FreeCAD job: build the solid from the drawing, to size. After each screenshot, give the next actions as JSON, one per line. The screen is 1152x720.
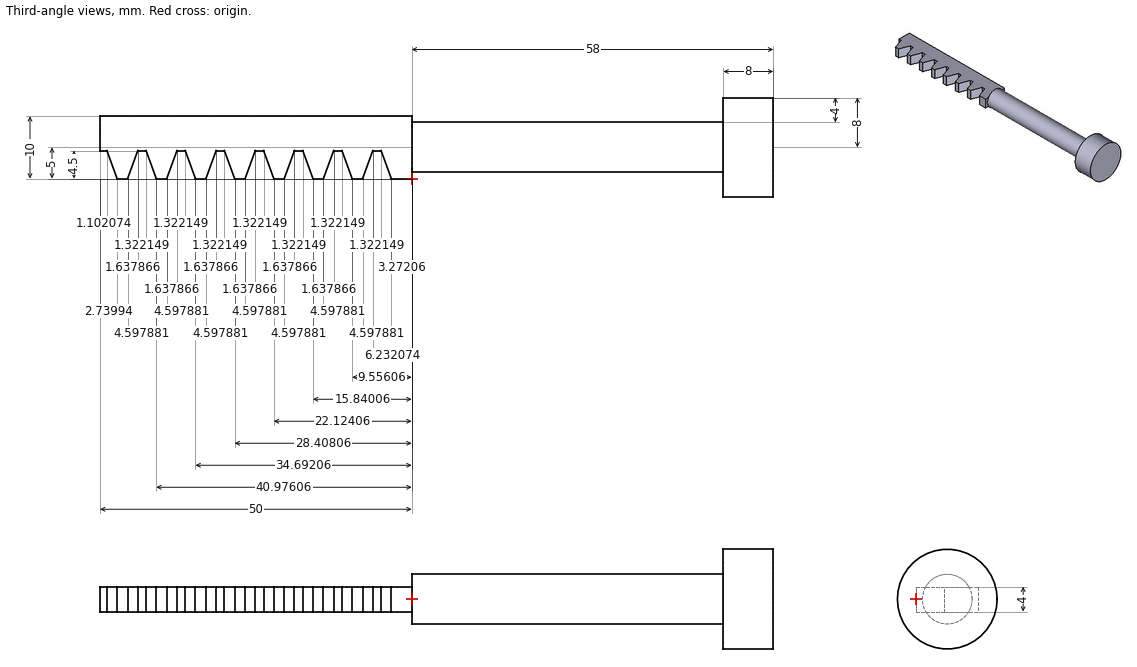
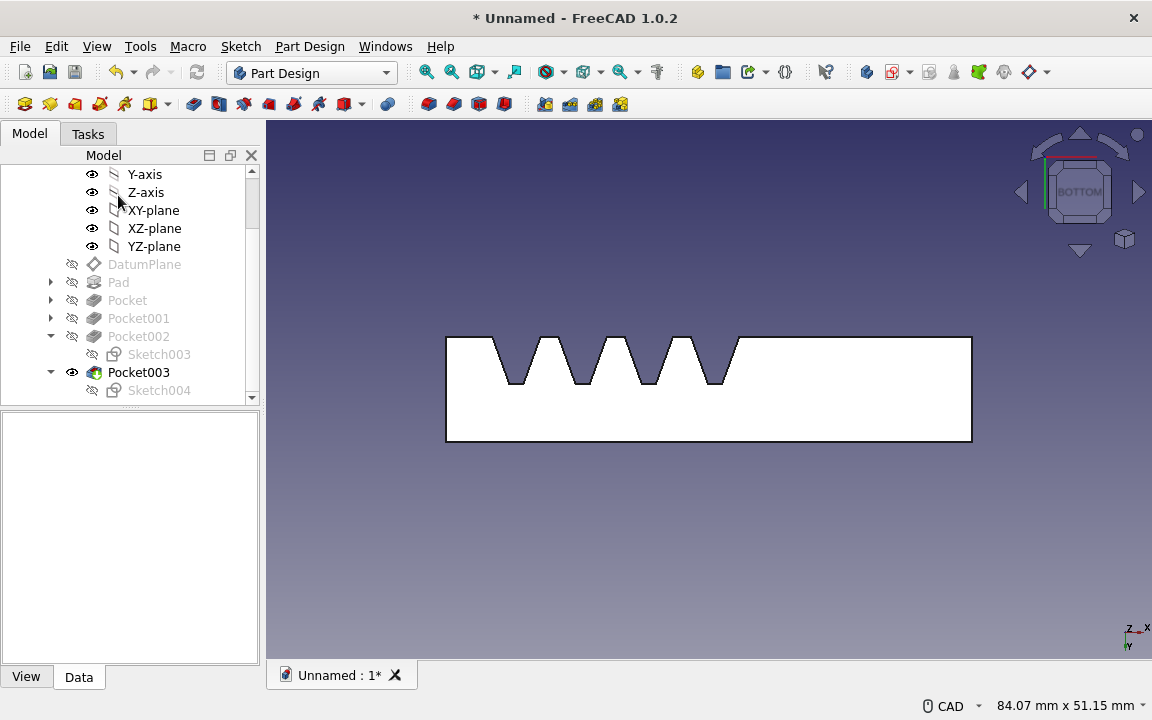
{"action": "left_click", "coordinate": [860, 389]}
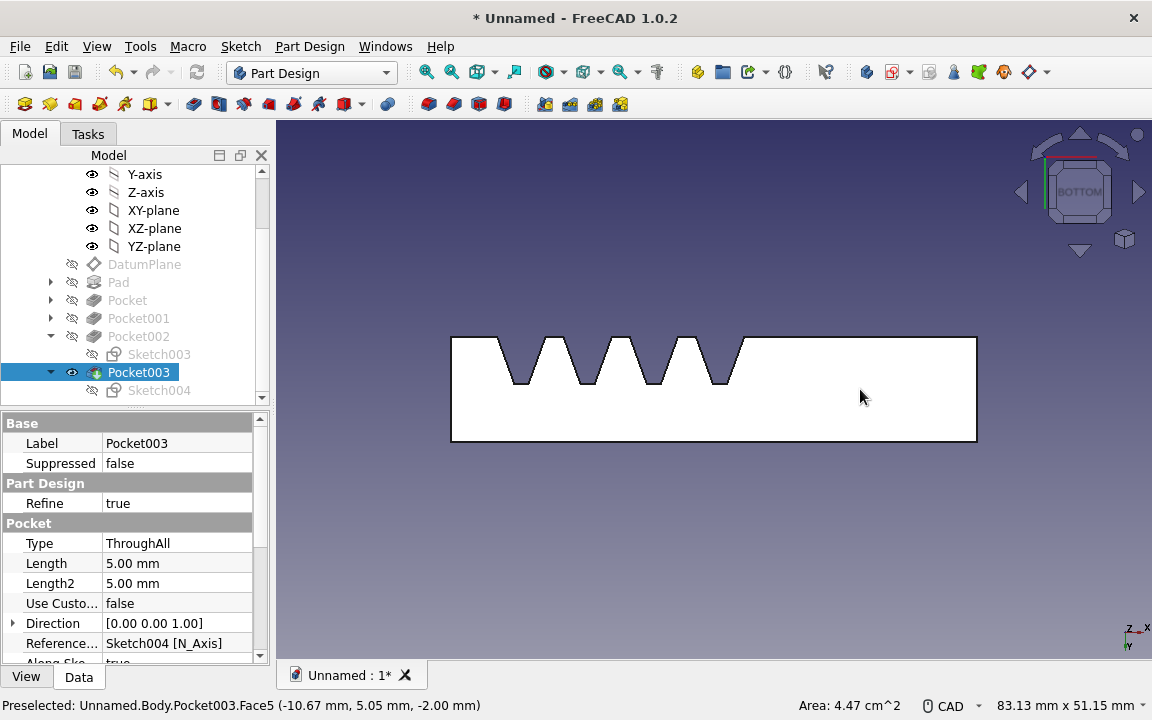
{"action": "left_click", "coordinate": [892, 72]}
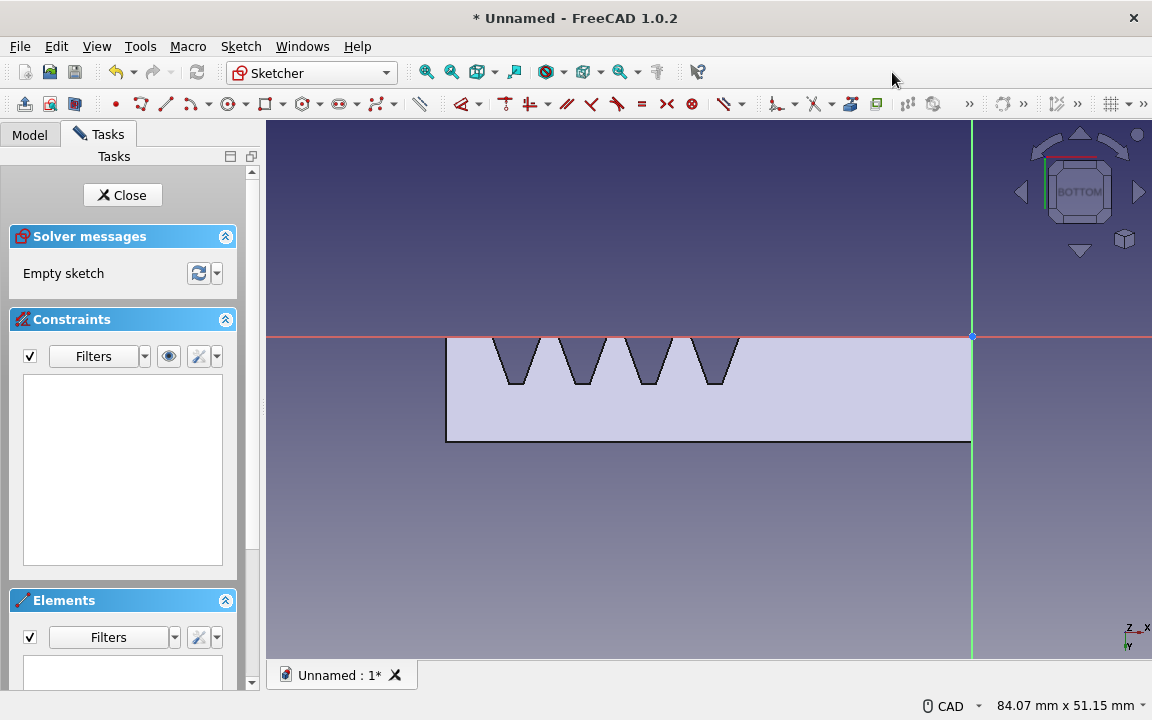
{"action": "scroll", "coordinate": [803, 356], "scroll_direction": "up", "scroll_amount": 10}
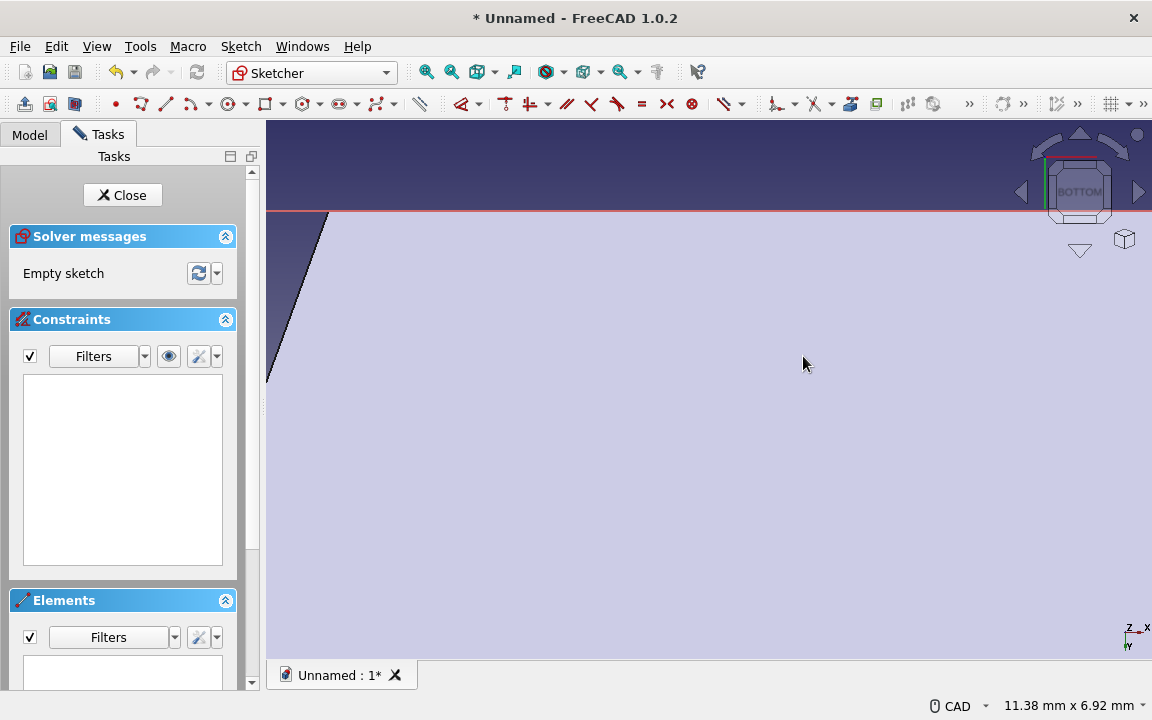
{"action": "left_click", "coordinate": [141, 104]}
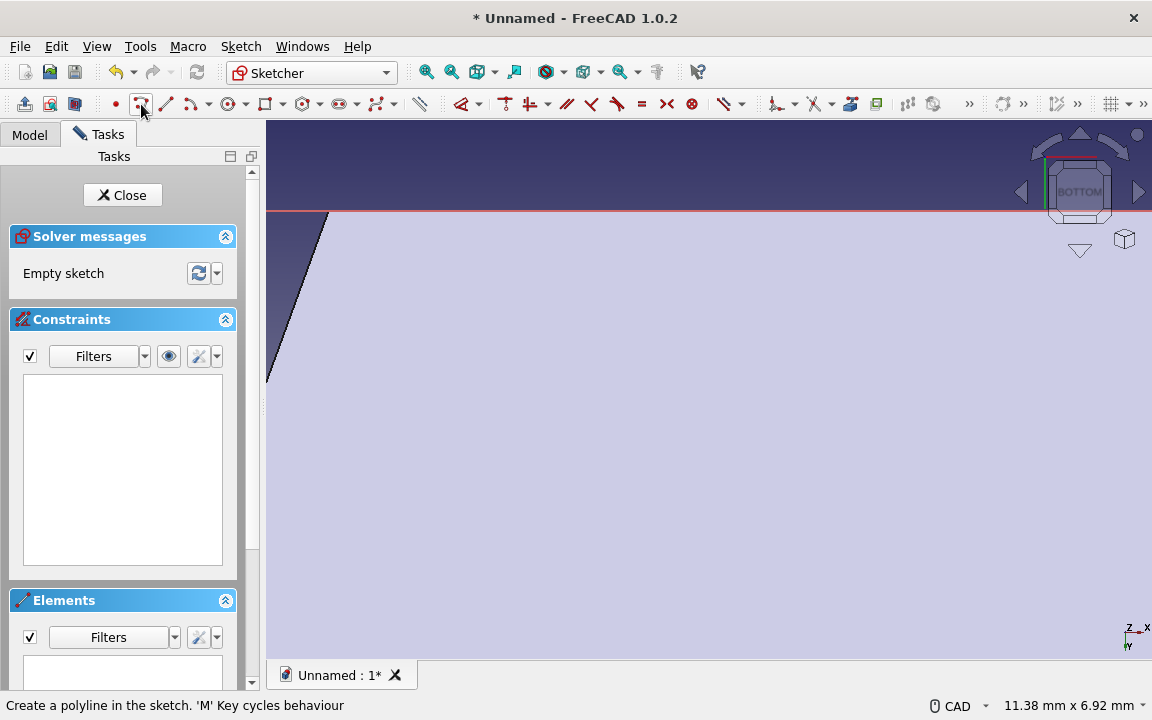
{"action": "left_click", "coordinate": [818, 211]}
{"action": "left_click", "coordinate": [460, 220]}
{"action": "left_click", "coordinate": [587, 562]}
{"action": "left_click", "coordinate": [690, 562]}
{"action": "left_click", "coordinate": [818, 211]}
{"action": "key", "text": "Escape"}
{"action": "key", "text": "Escape"}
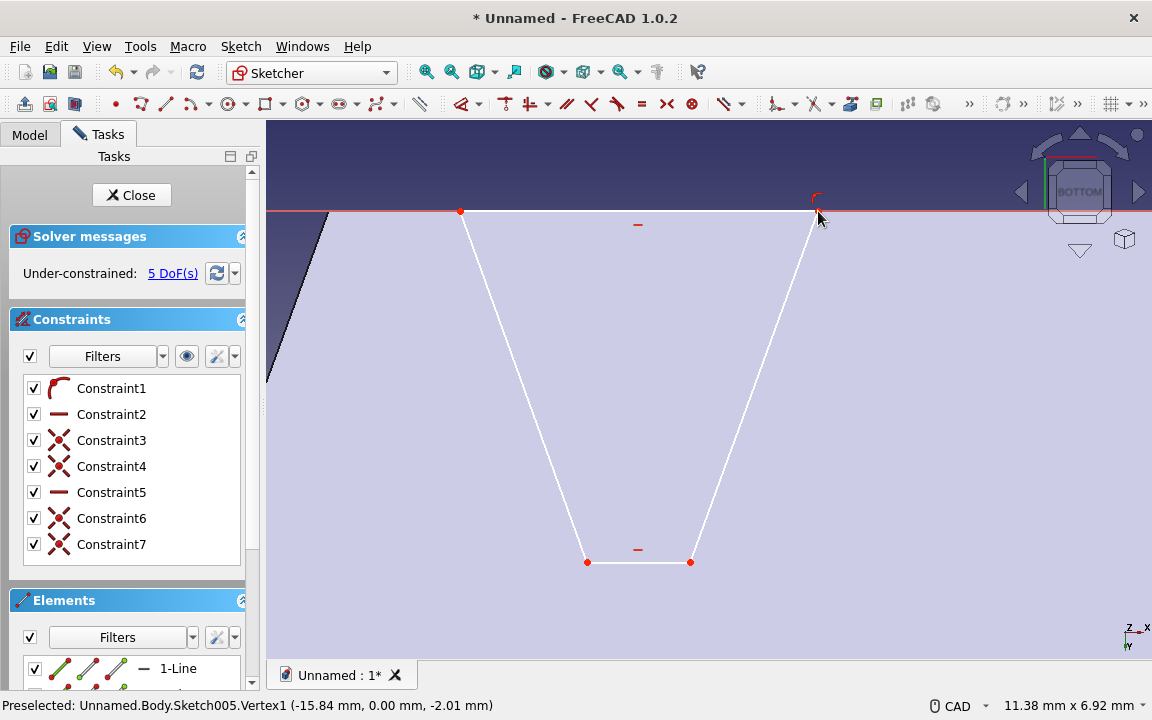
{"action": "left_click", "coordinate": [460, 104]}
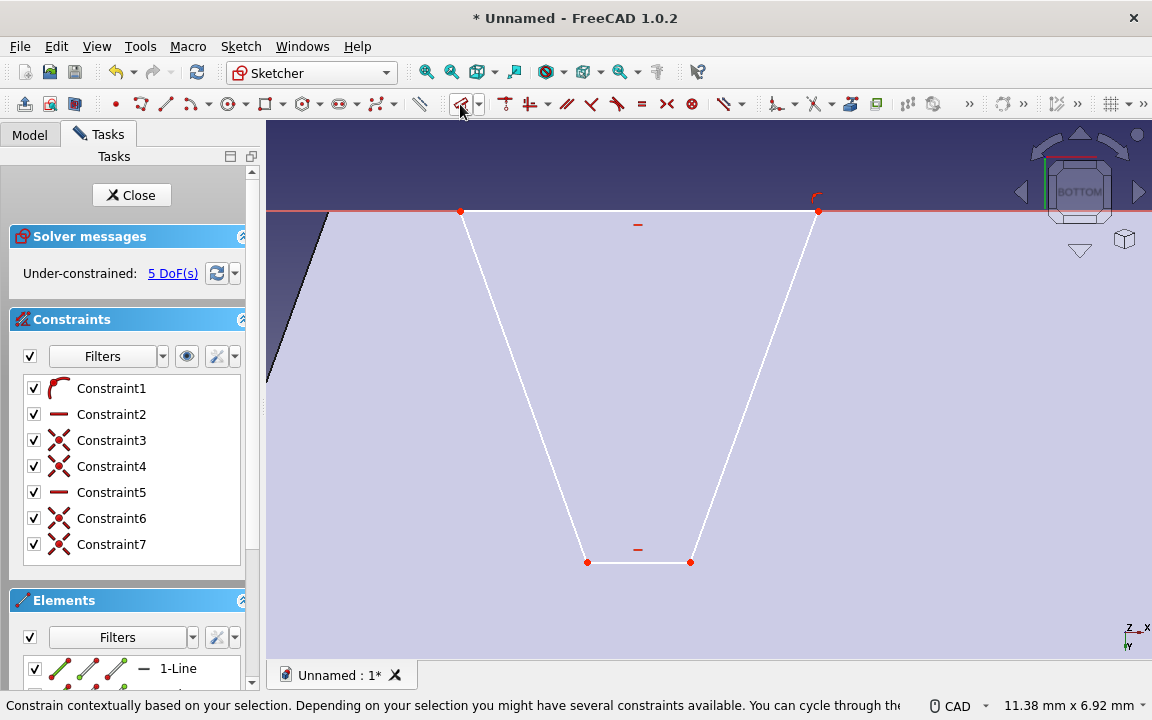
{"action": "left_click", "coordinate": [587, 563]}
{"action": "left_click", "coordinate": [553, 387]}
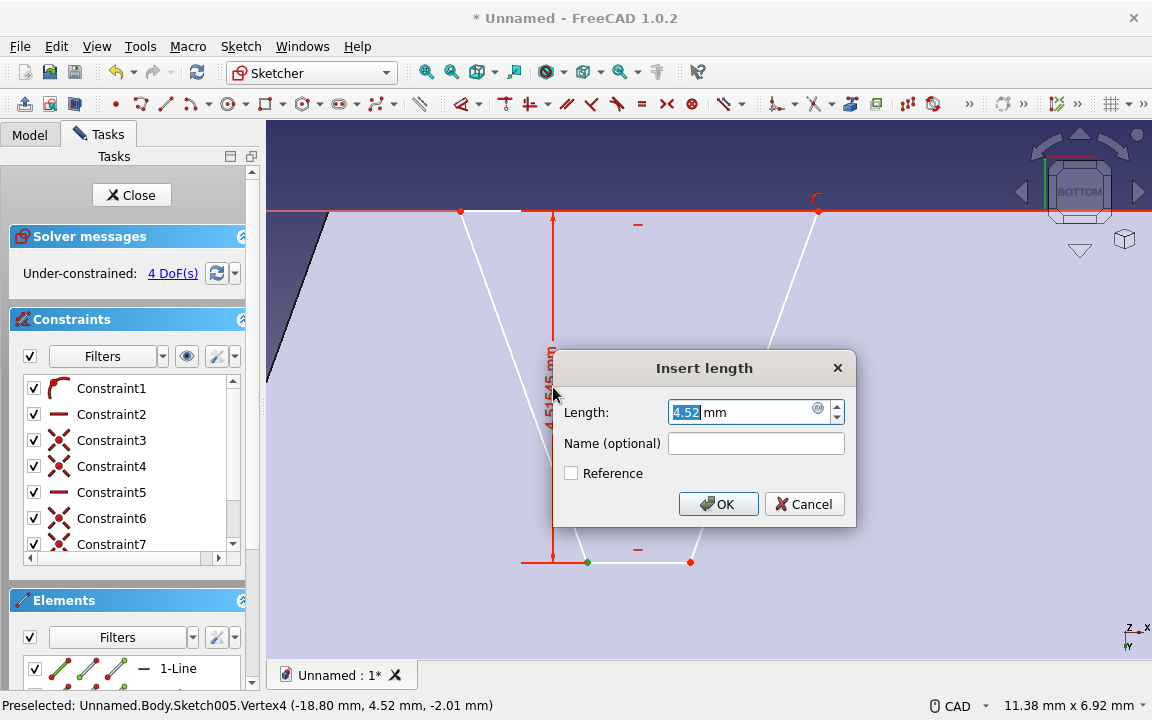
{"action": "type", "text": "4.5"}
{"action": "key", "text": "Return"}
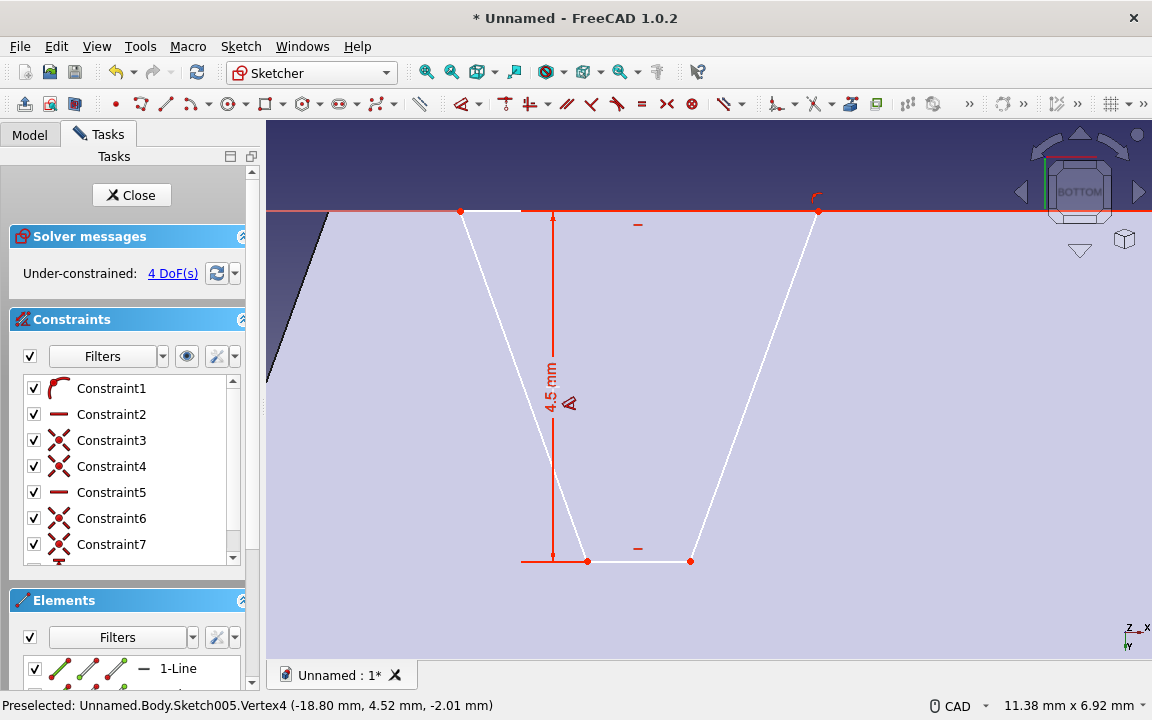
{"action": "left_click", "coordinate": [711, 211]}
{"action": "left_click", "coordinate": [639, 177]}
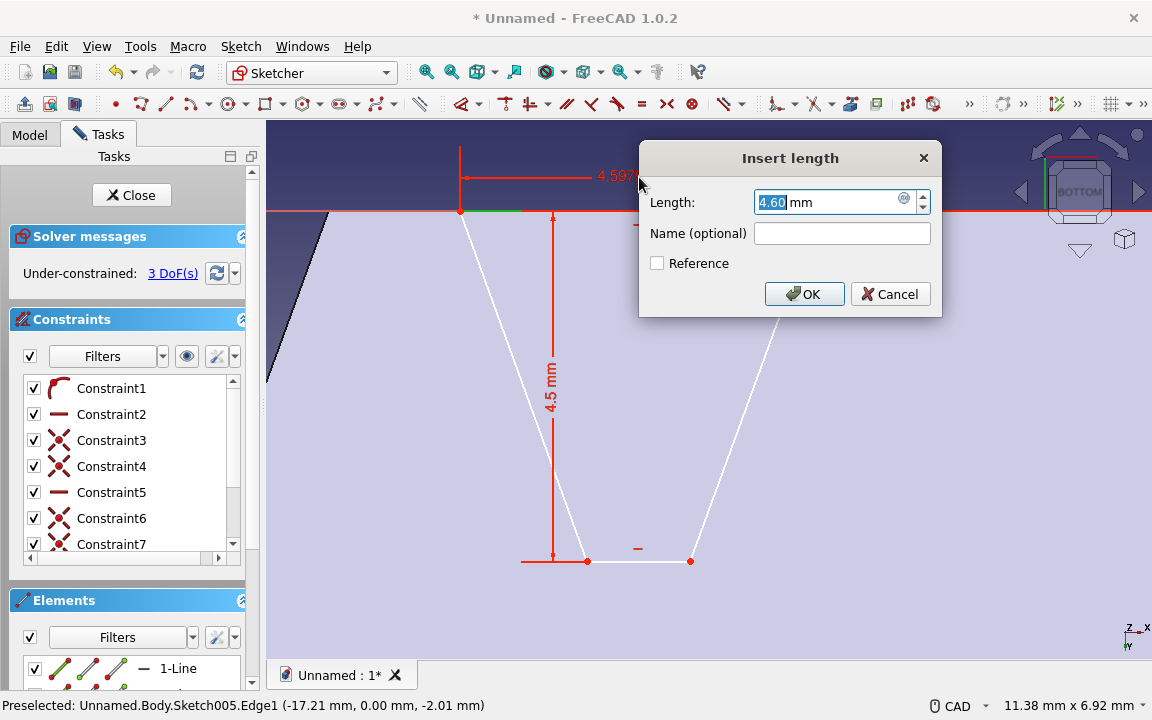
{"action": "type", "text": "4.597881"}
{"action": "key", "text": "Return"}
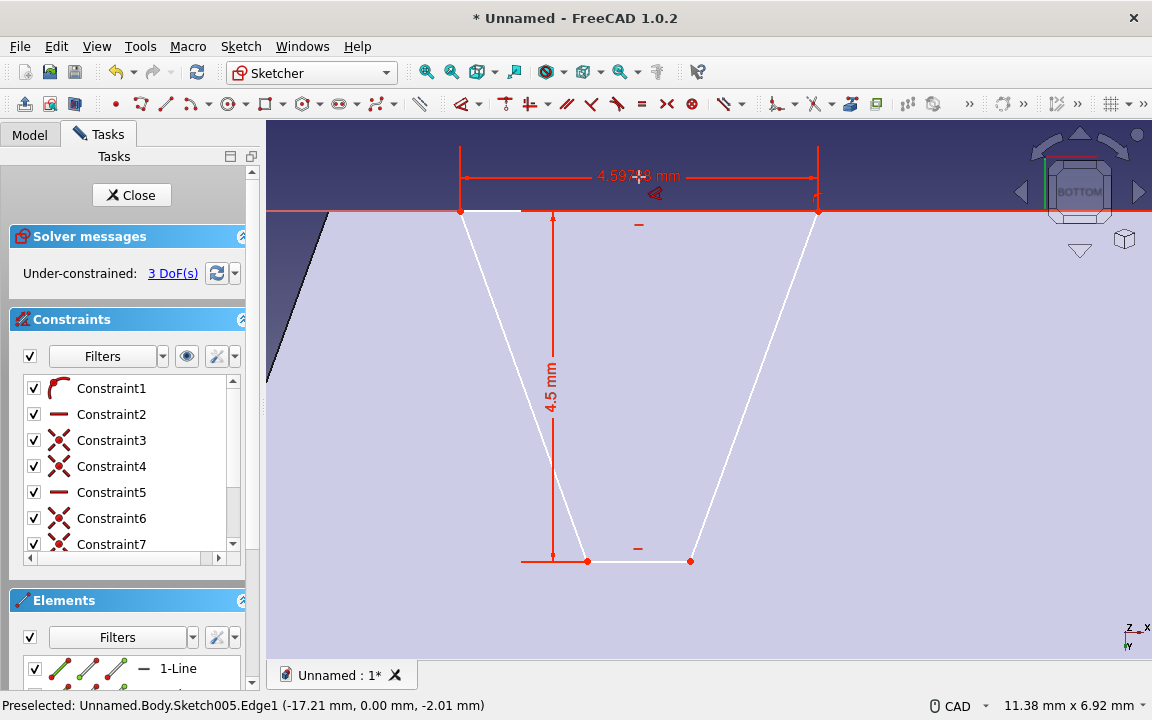
{"action": "left_click", "coordinate": [618, 562]}
{"action": "left_click", "coordinate": [638, 596]}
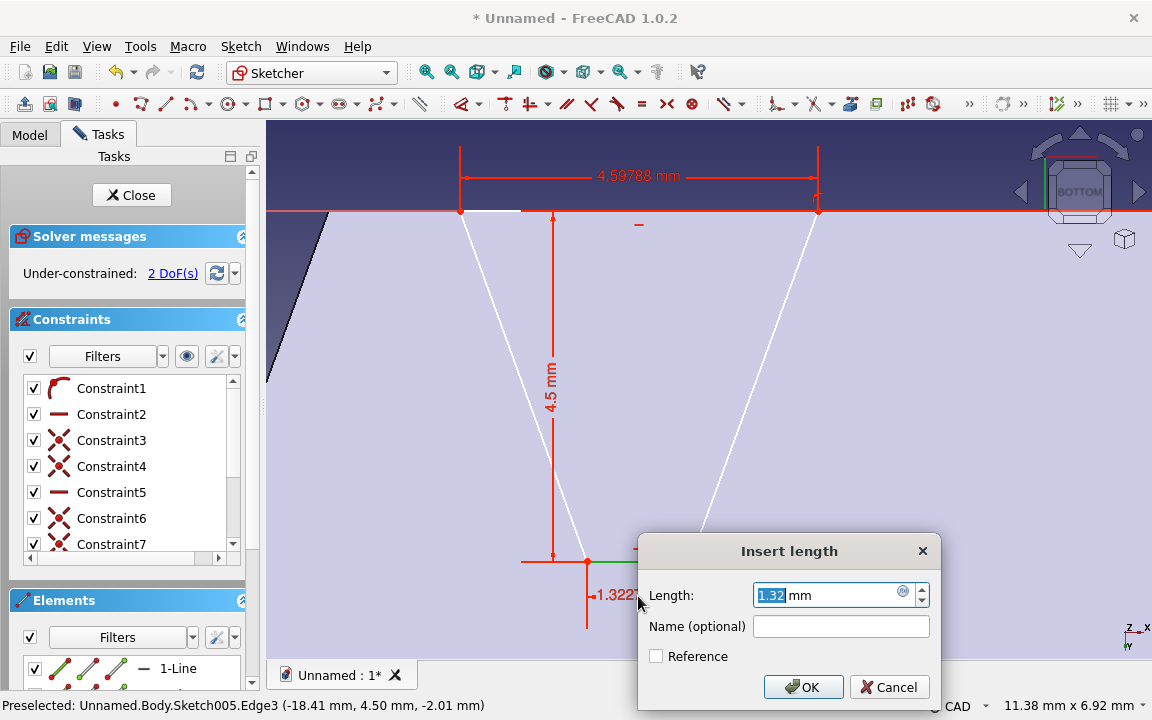
{"action": "type", "text": "1.322149"}
{"action": "key", "text": "Return"}